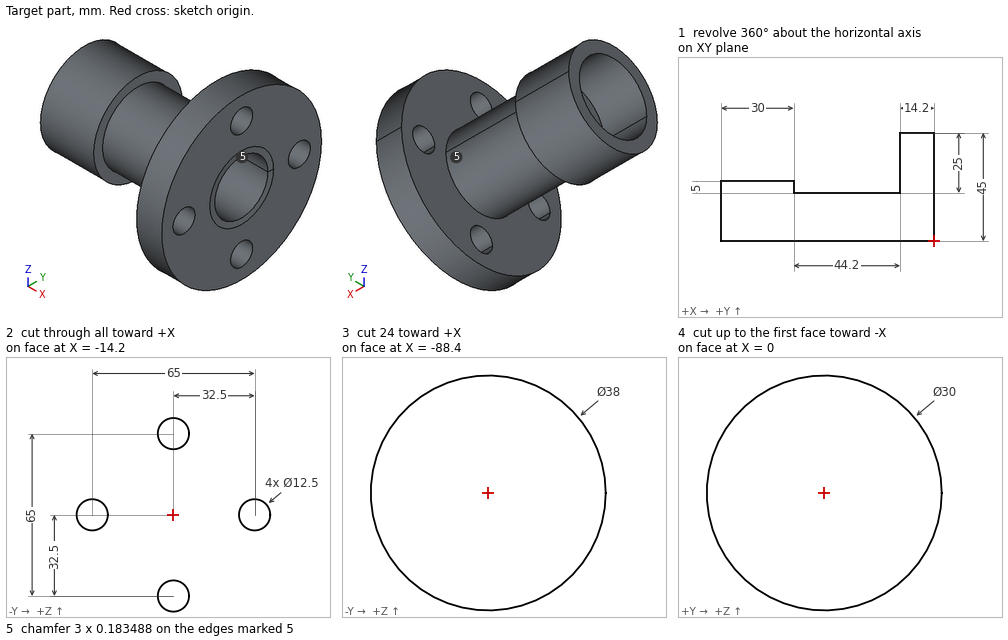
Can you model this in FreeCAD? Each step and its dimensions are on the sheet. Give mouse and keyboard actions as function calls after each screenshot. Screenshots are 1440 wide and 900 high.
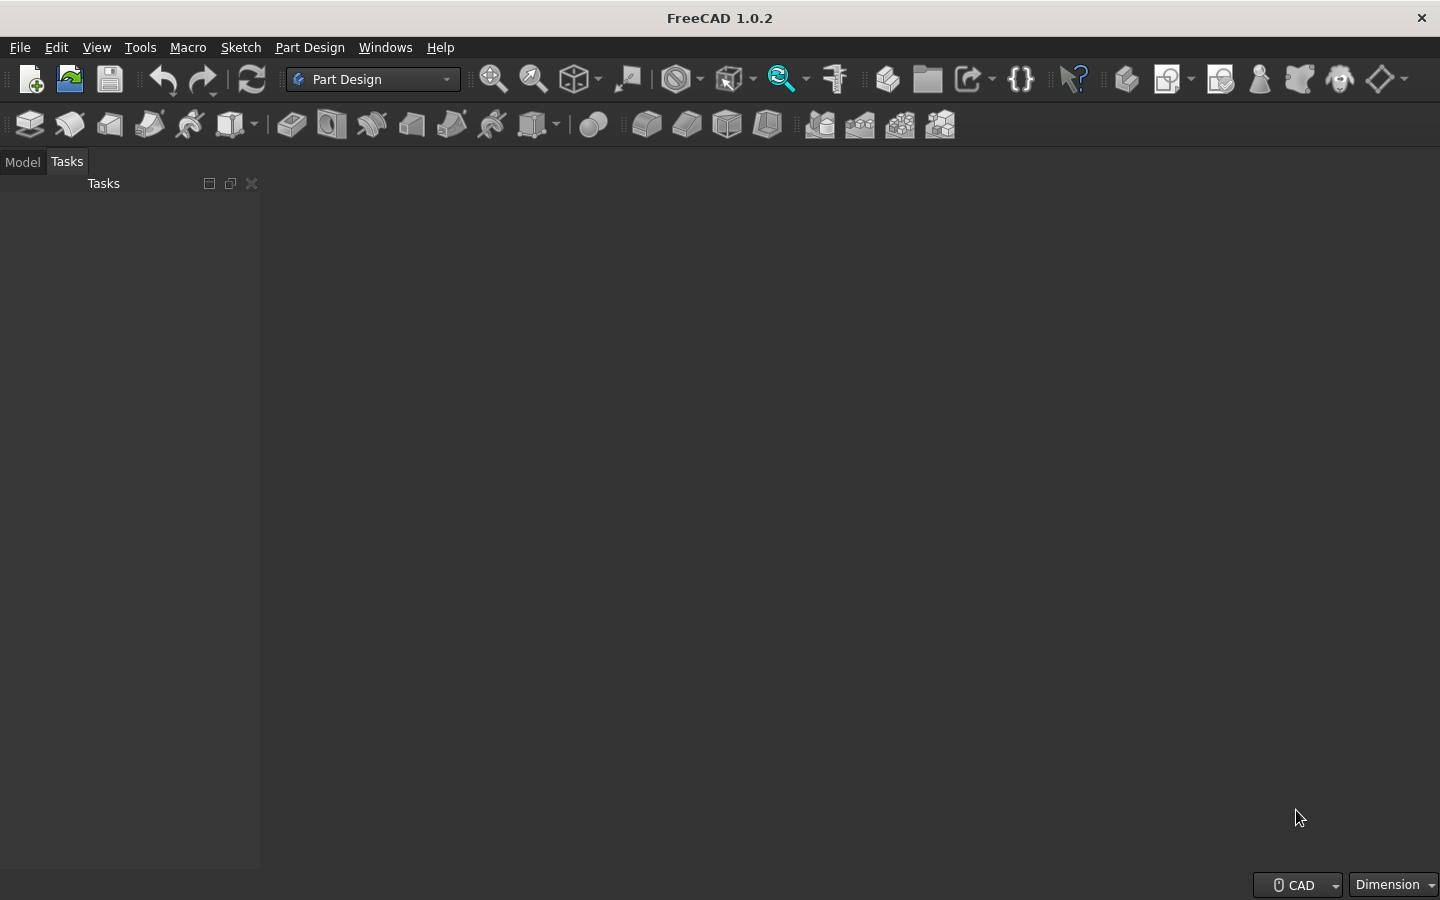
key(ctrl+n)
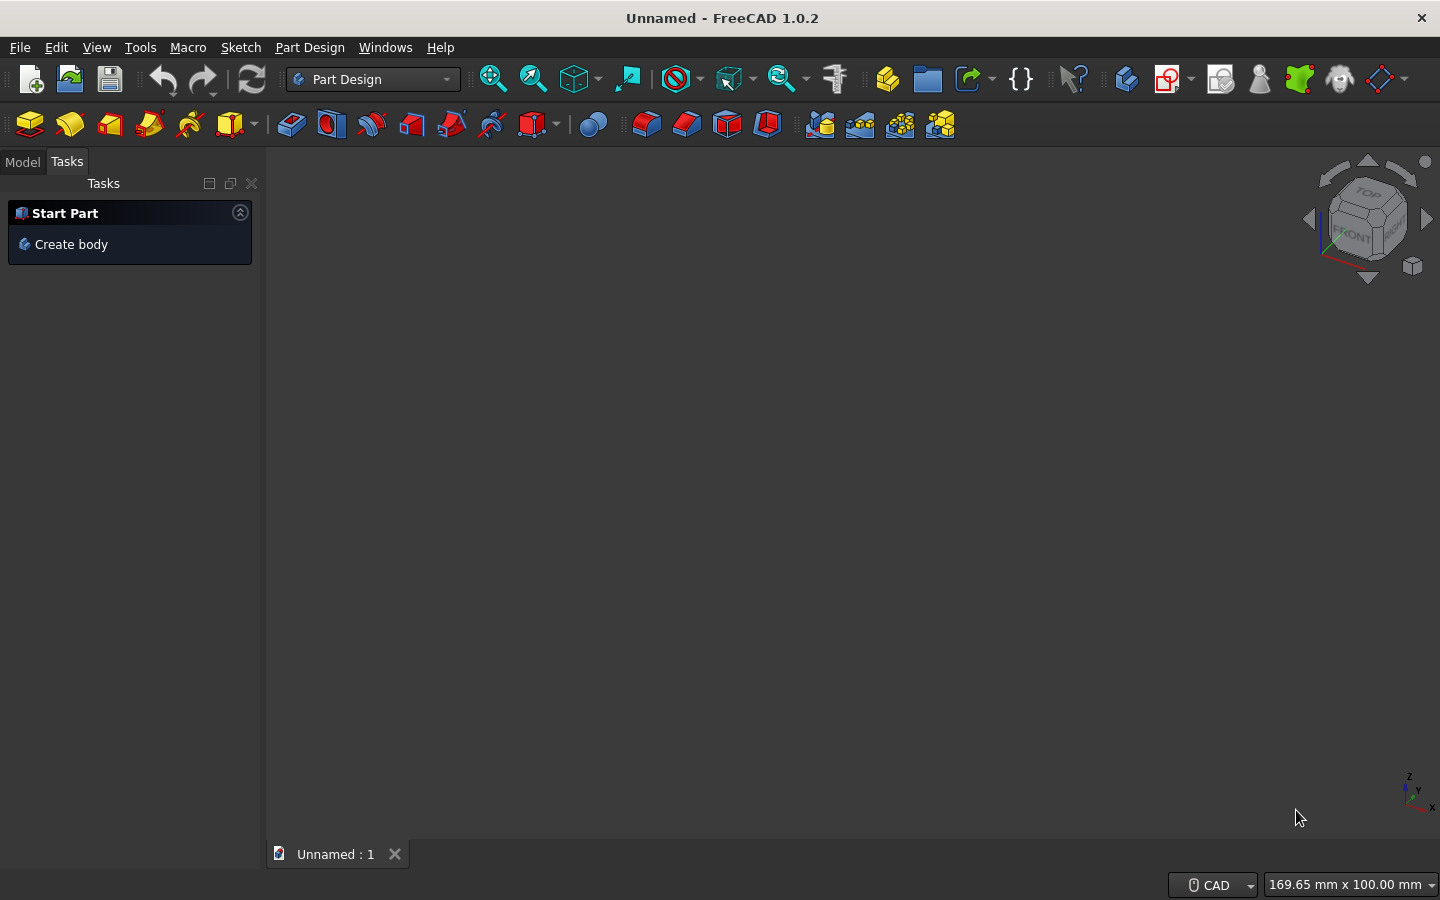
click(1168, 80)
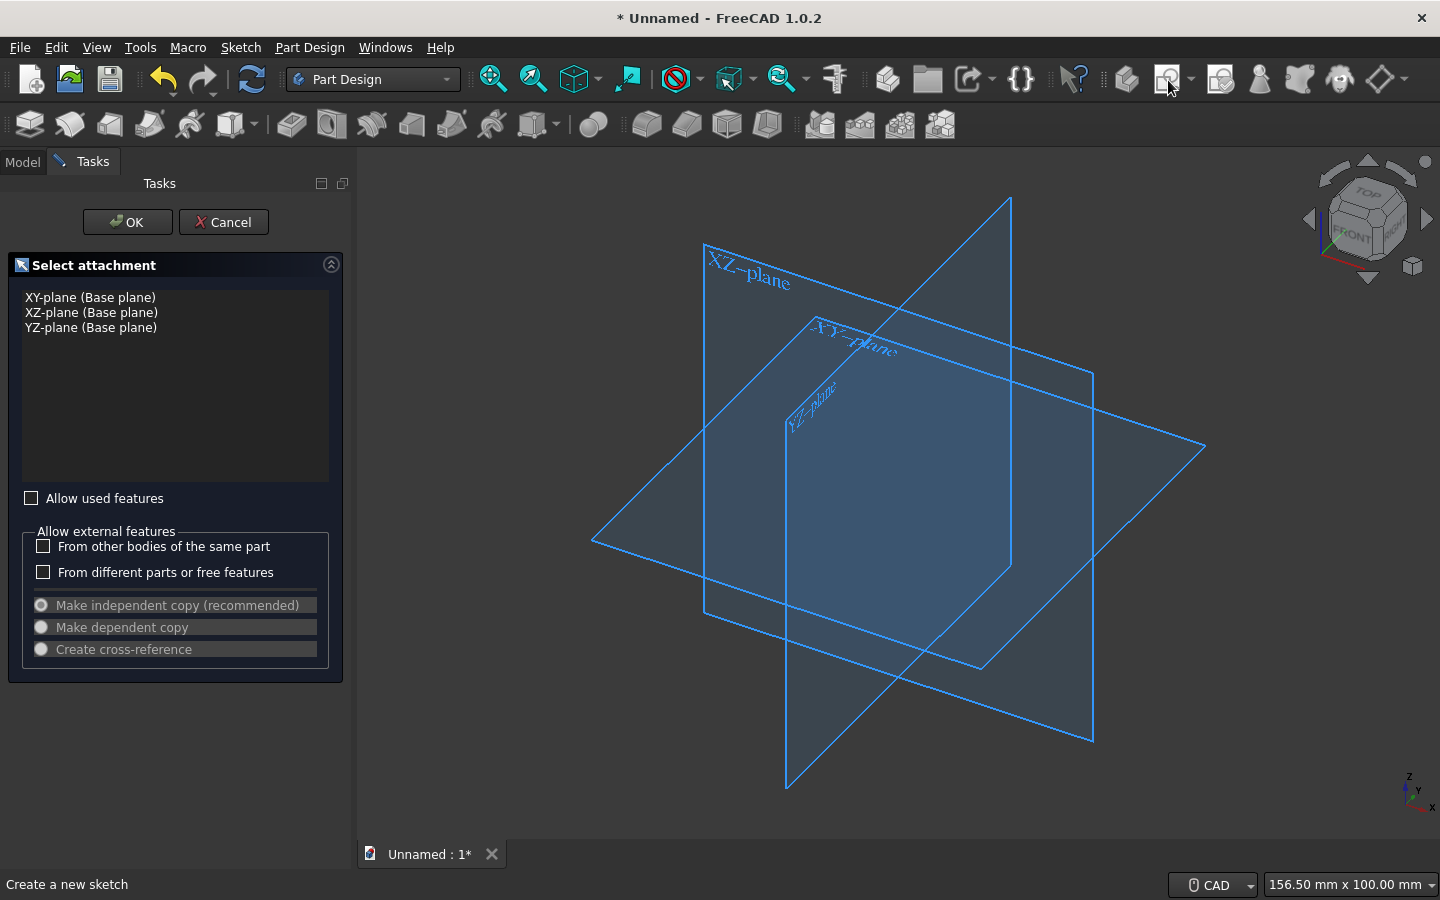
click(82, 298)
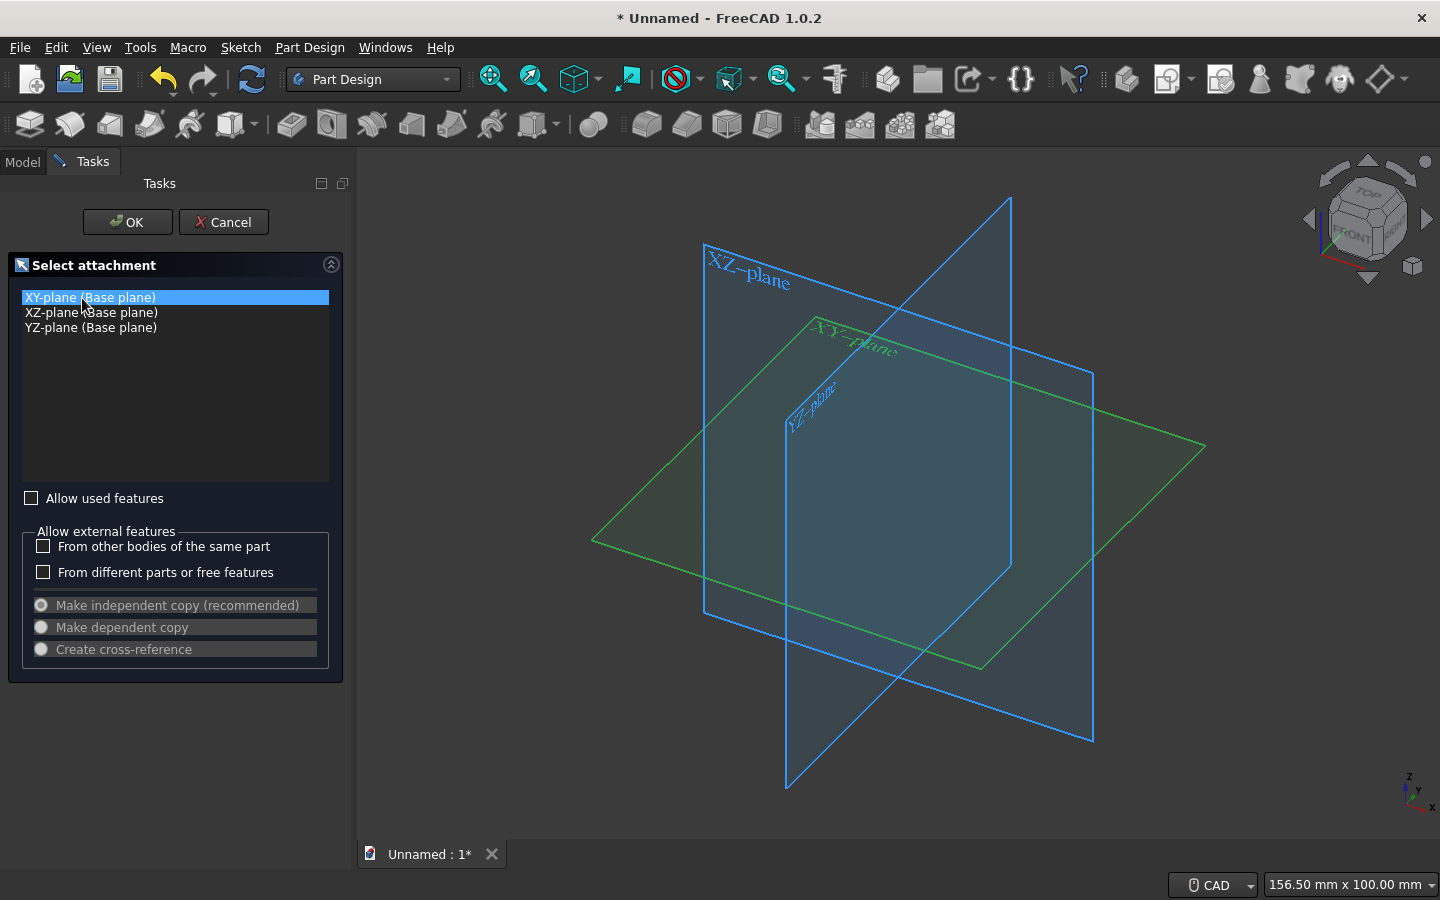
click(128, 222)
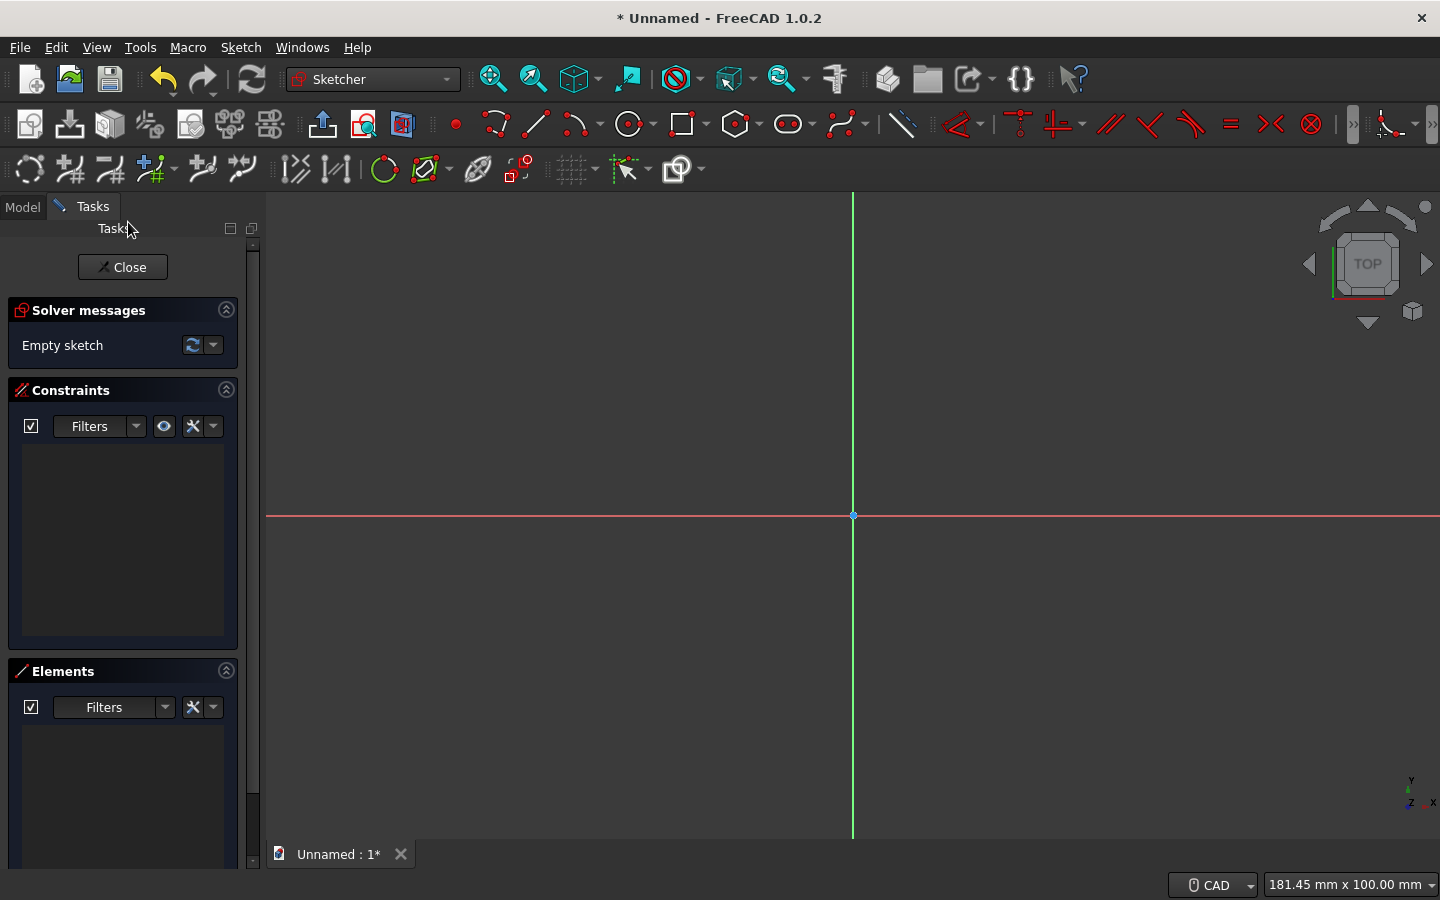
scroll(1275, 811, down, 1)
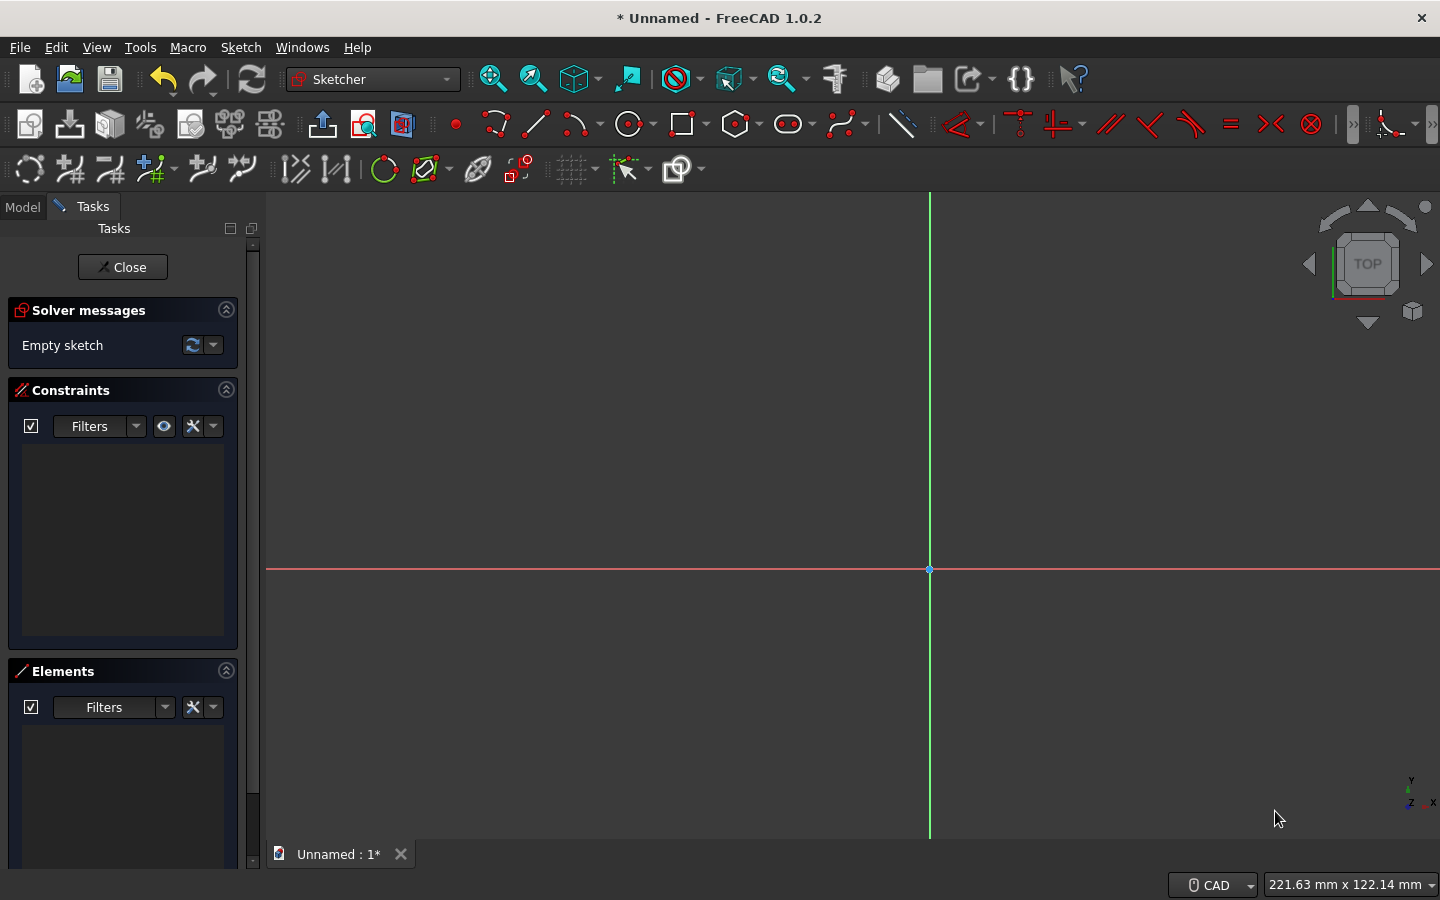
scroll(515, 317, up, 2)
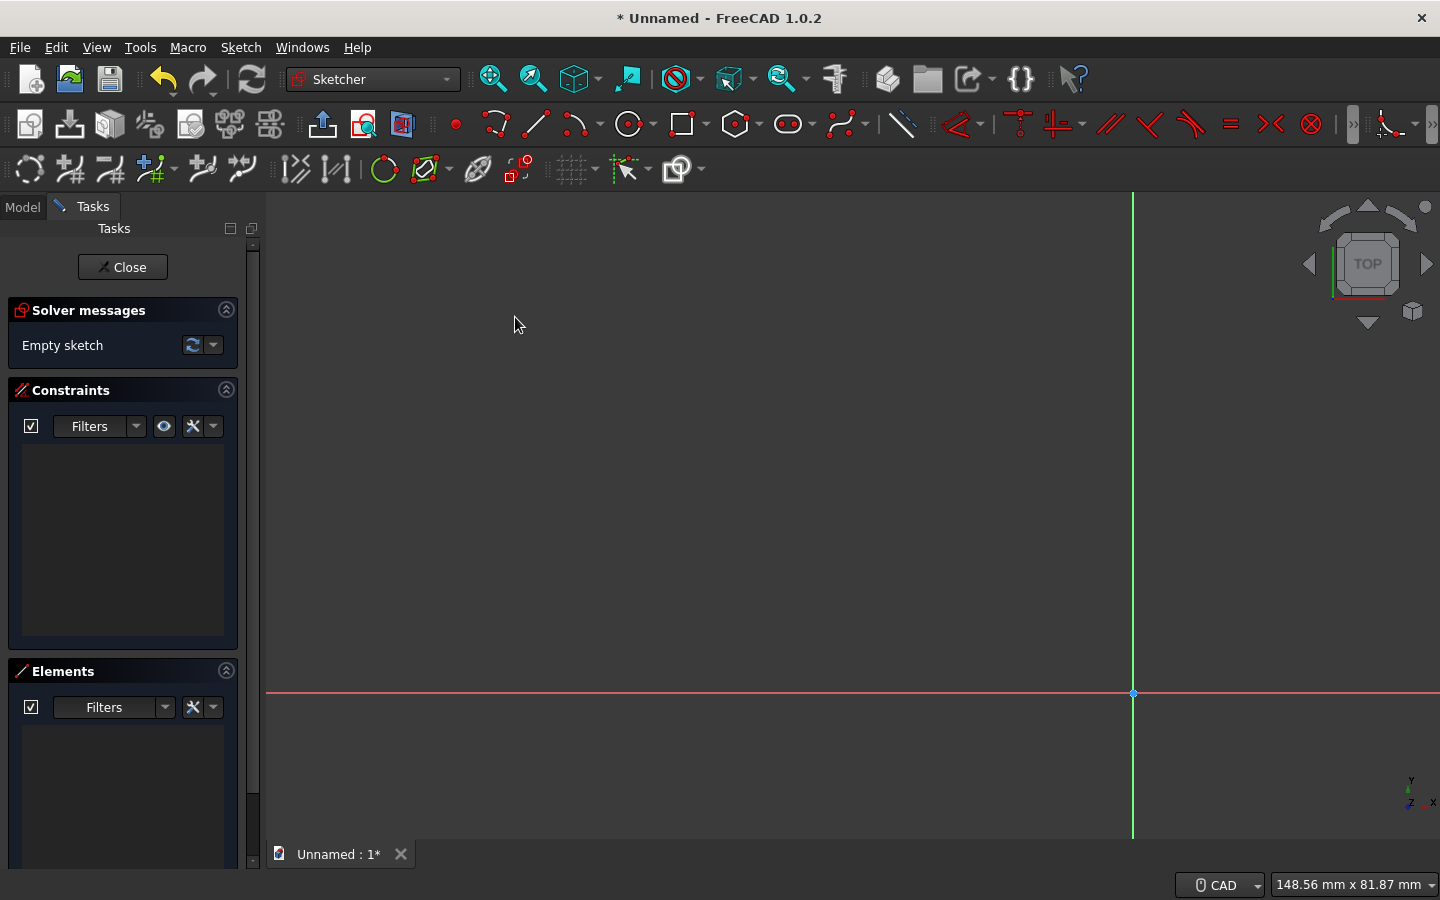
key(g)
key(m)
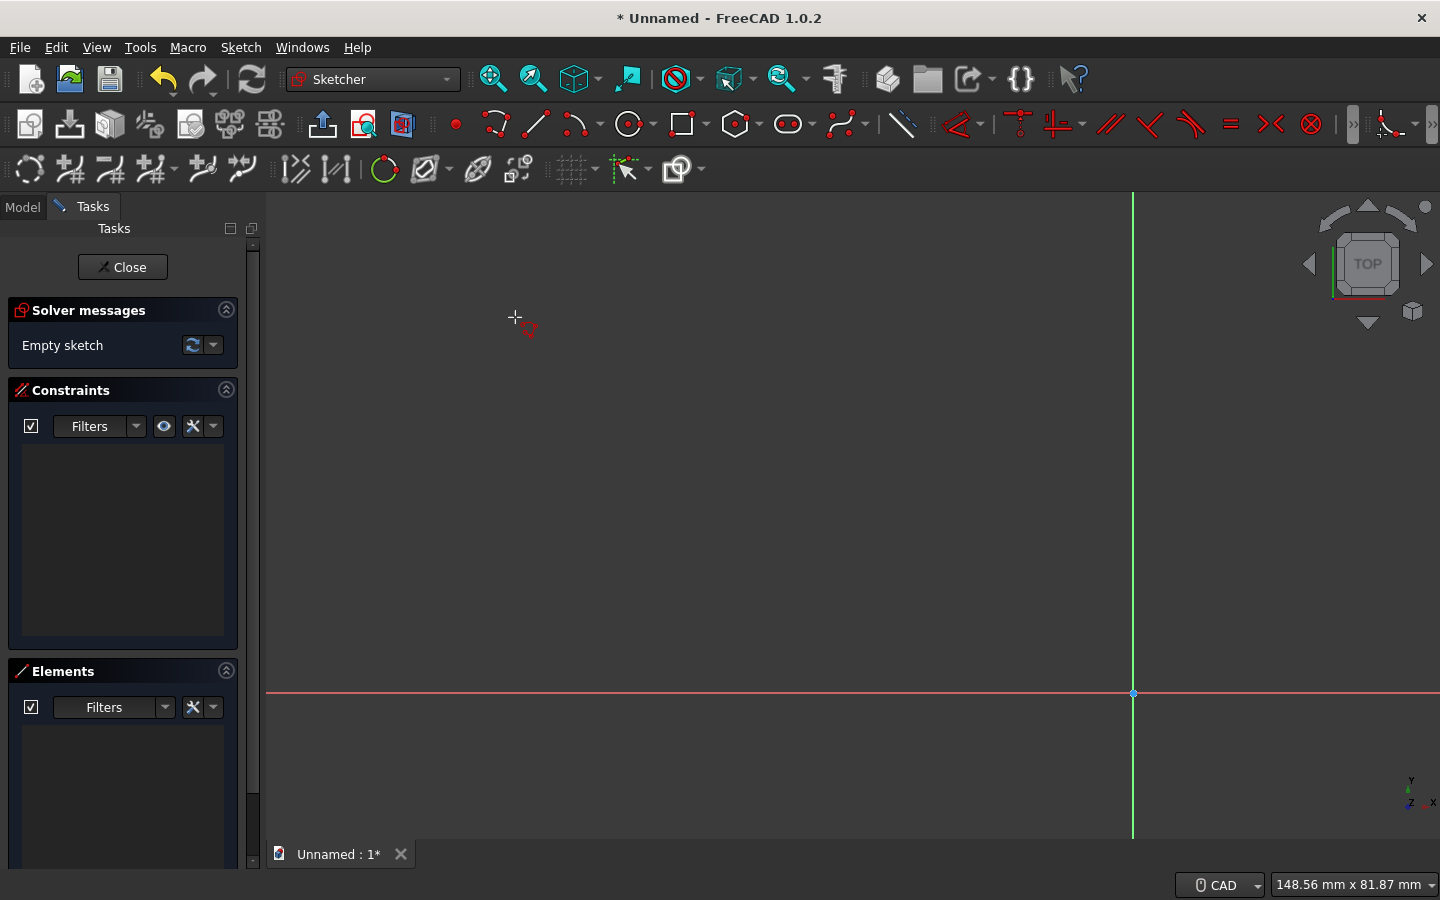
click(1133, 693)
click(1124, 338)
click(1021, 338)
click(1021, 535)
click(672, 535)
click(672, 496)
click(435, 496)
click(435, 684)
click(1133, 693)
key(Escape)
key(Escape)